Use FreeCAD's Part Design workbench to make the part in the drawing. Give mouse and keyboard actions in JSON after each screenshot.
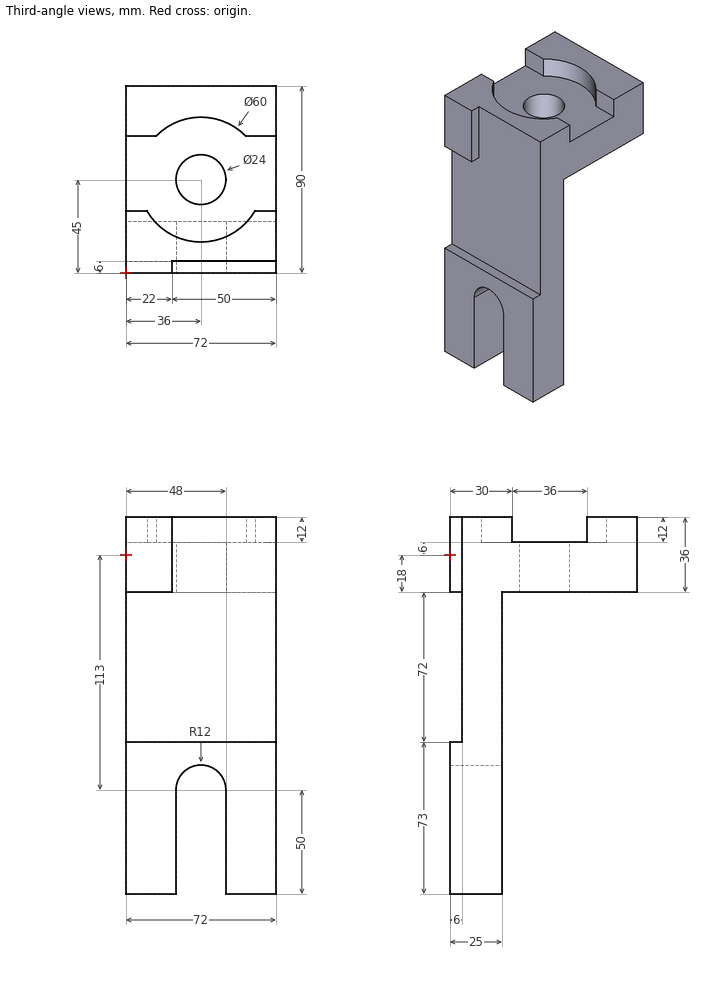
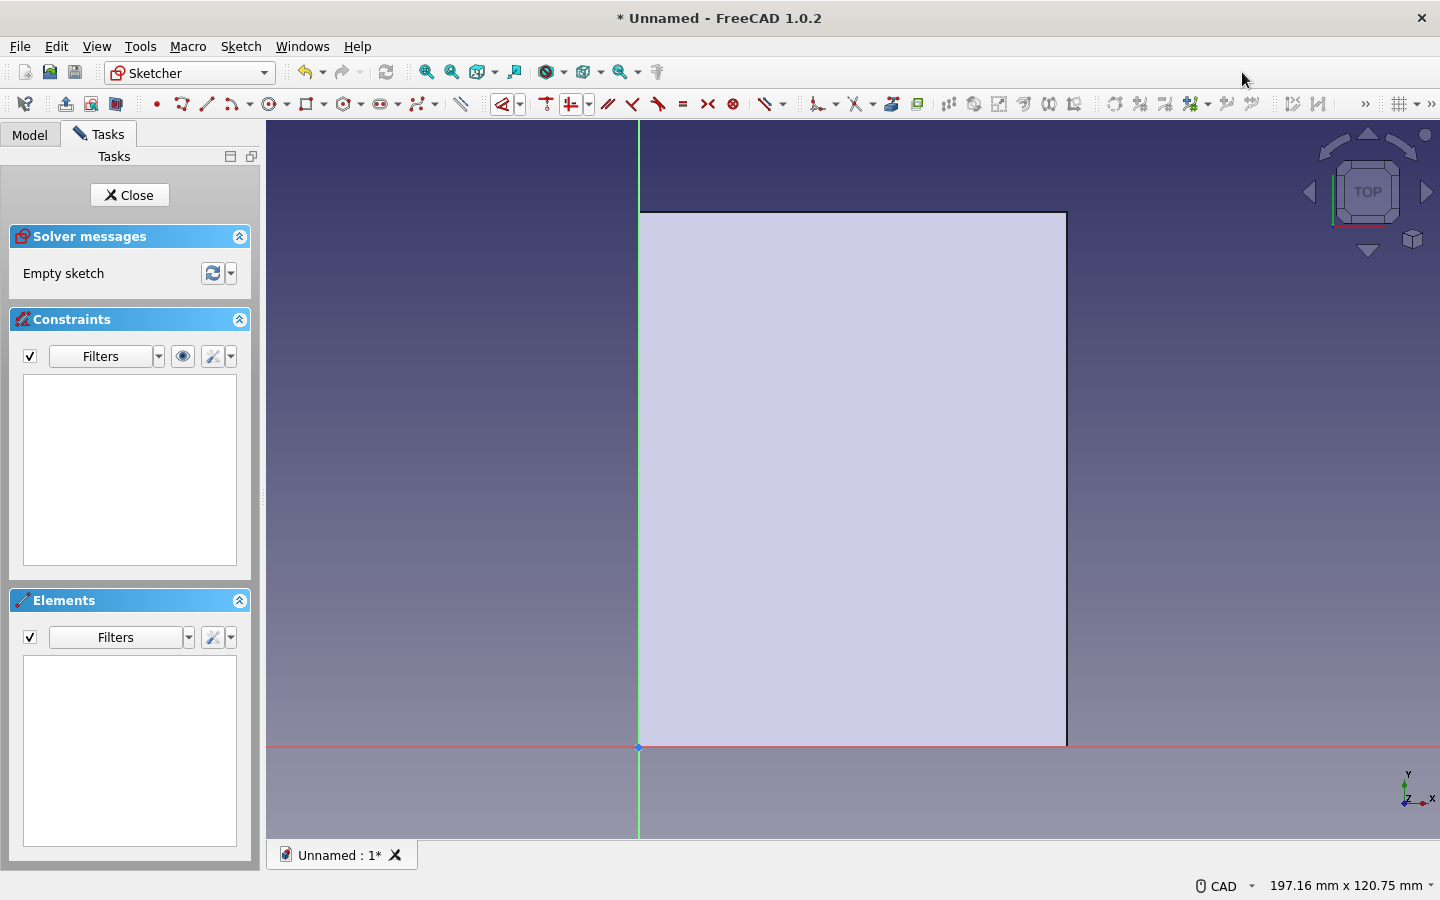
{"action": "key", "text": "g c"}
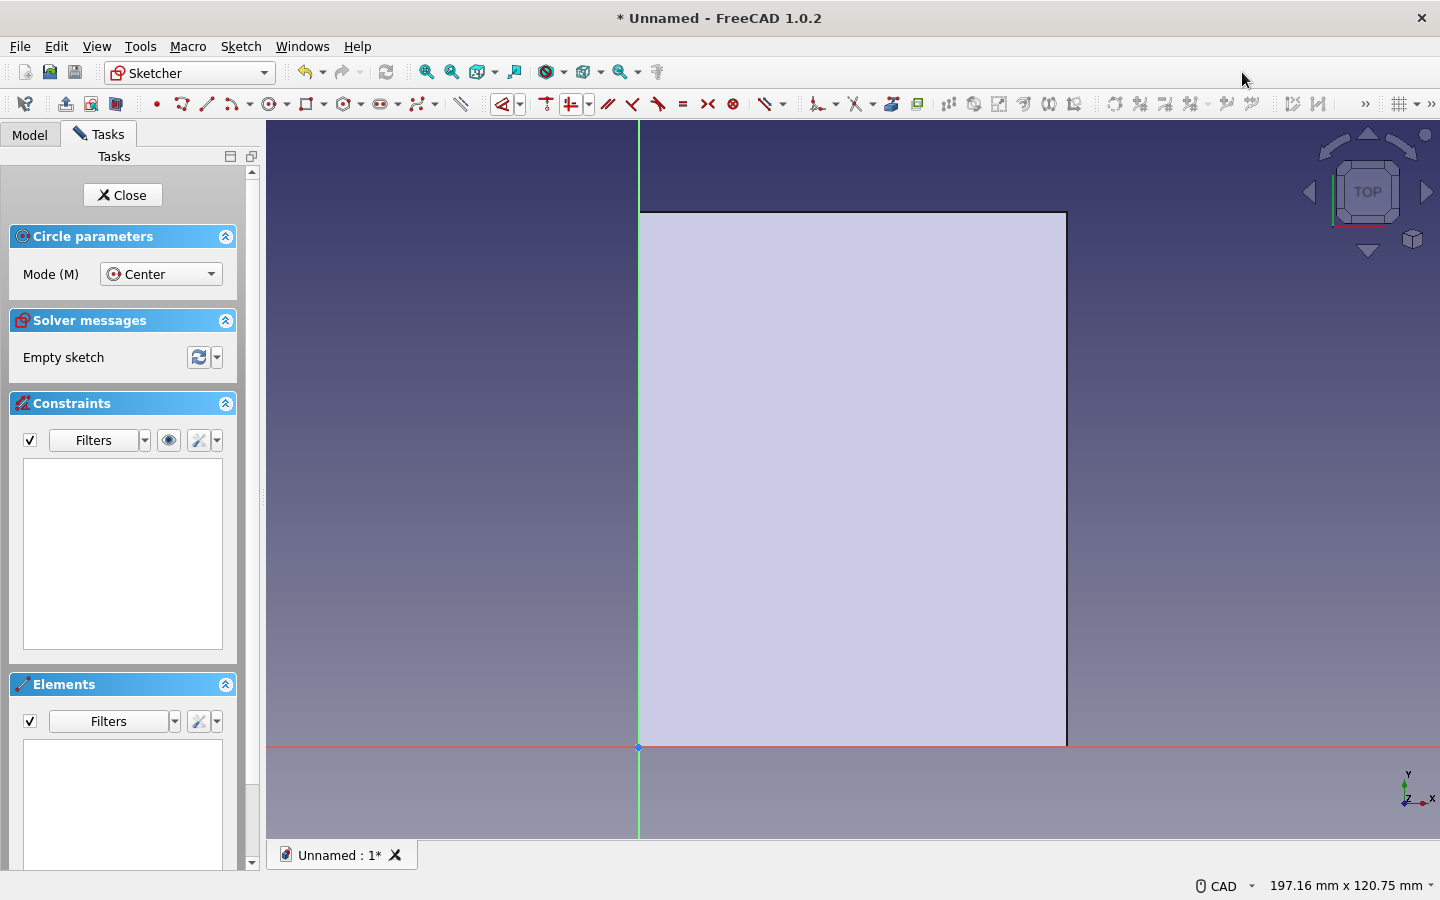
{"action": "left_click", "coordinate": [853, 480]}
{"action": "mouse_move", "coordinate": [979, 353]}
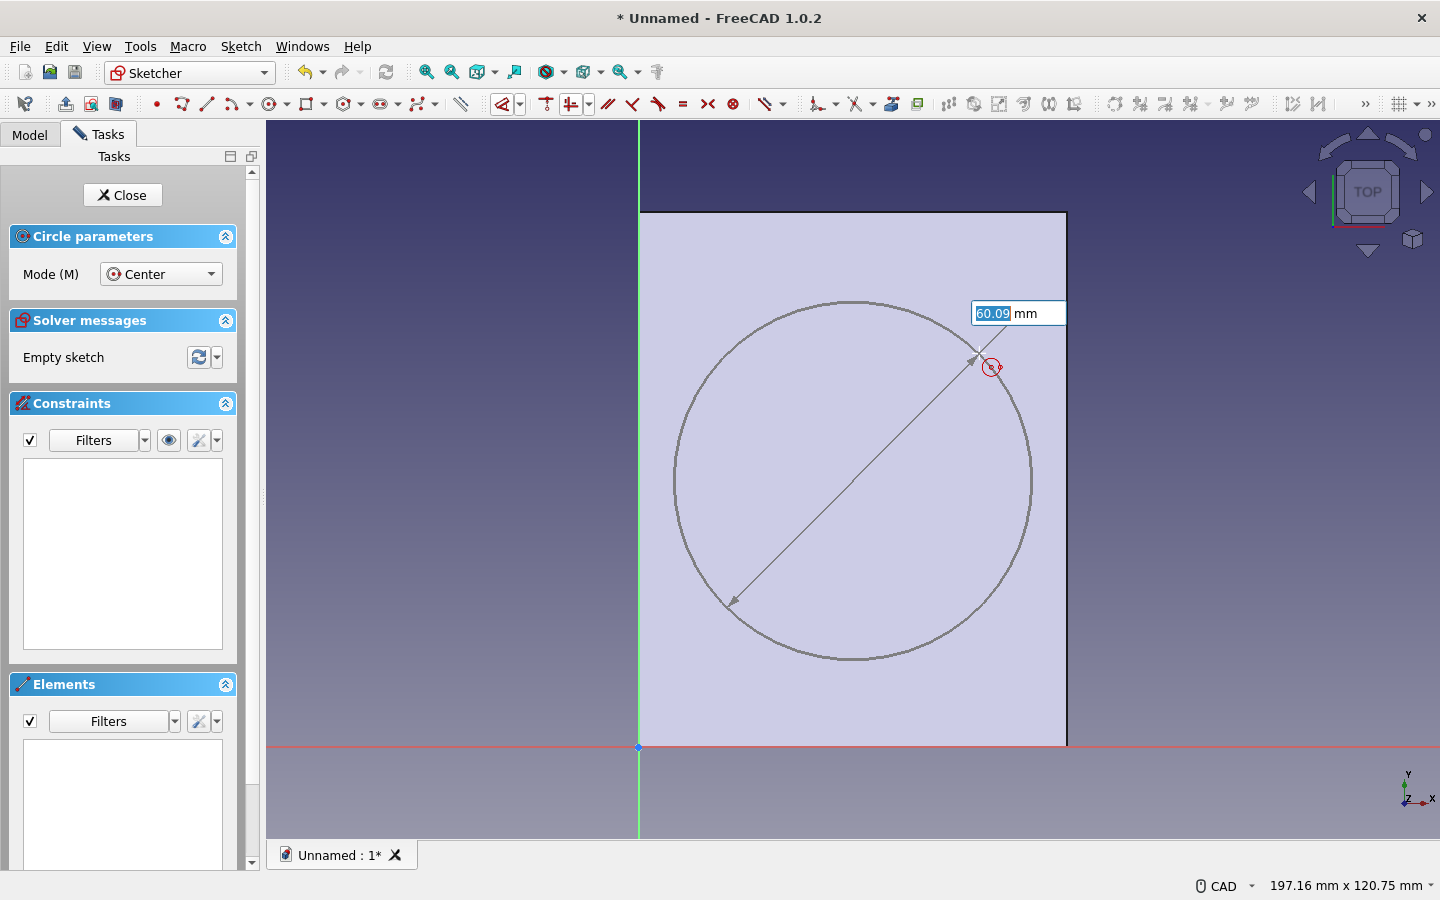
{"action": "type", "text": "60"}
{"action": "key", "text": "Return"}
{"action": "key", "text": "Escape"}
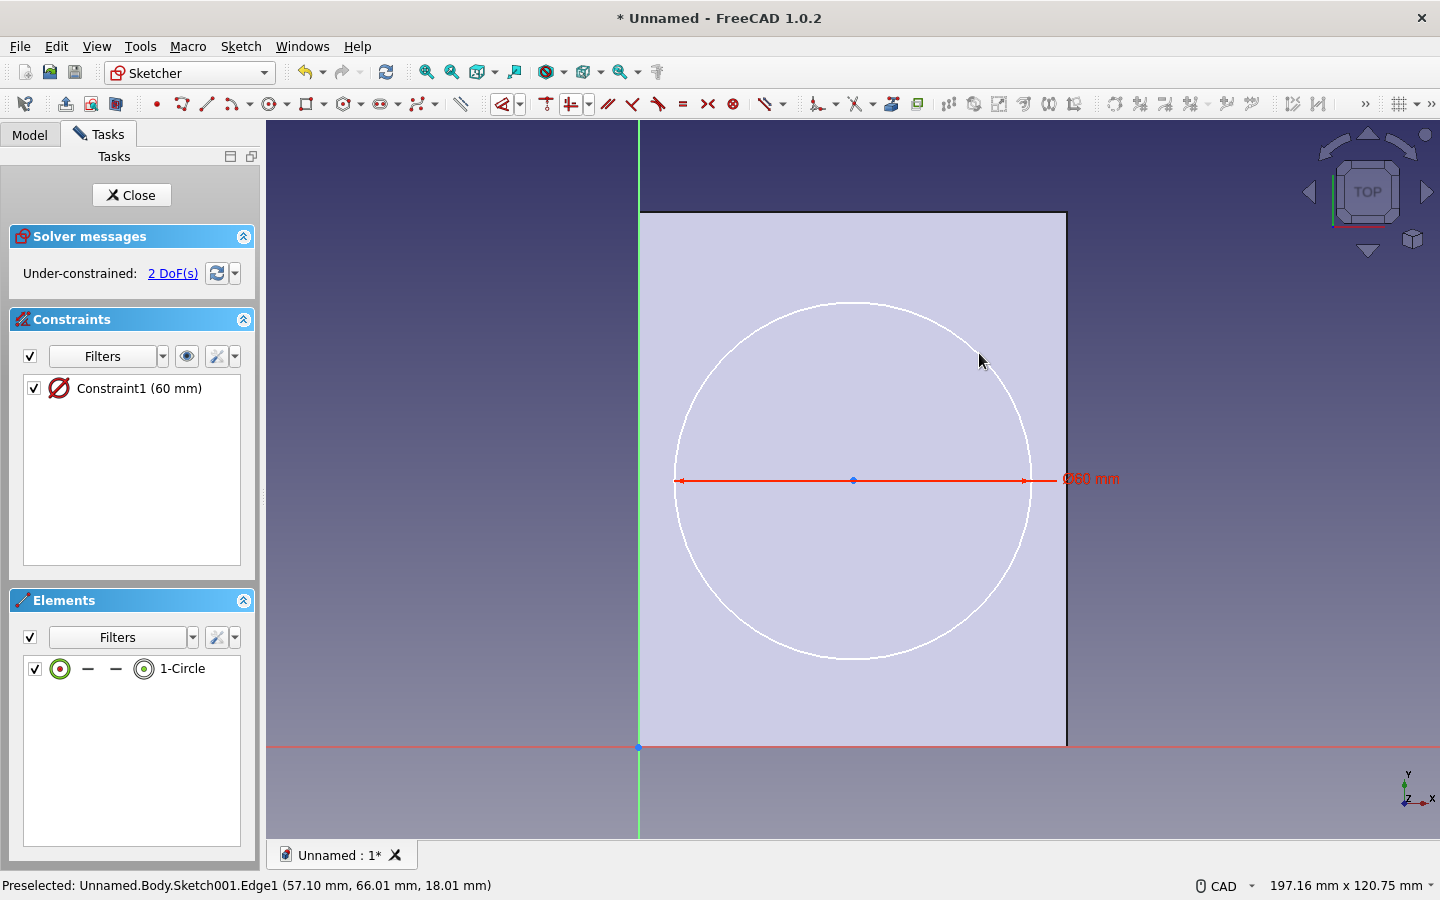
{"action": "key", "text": "d"}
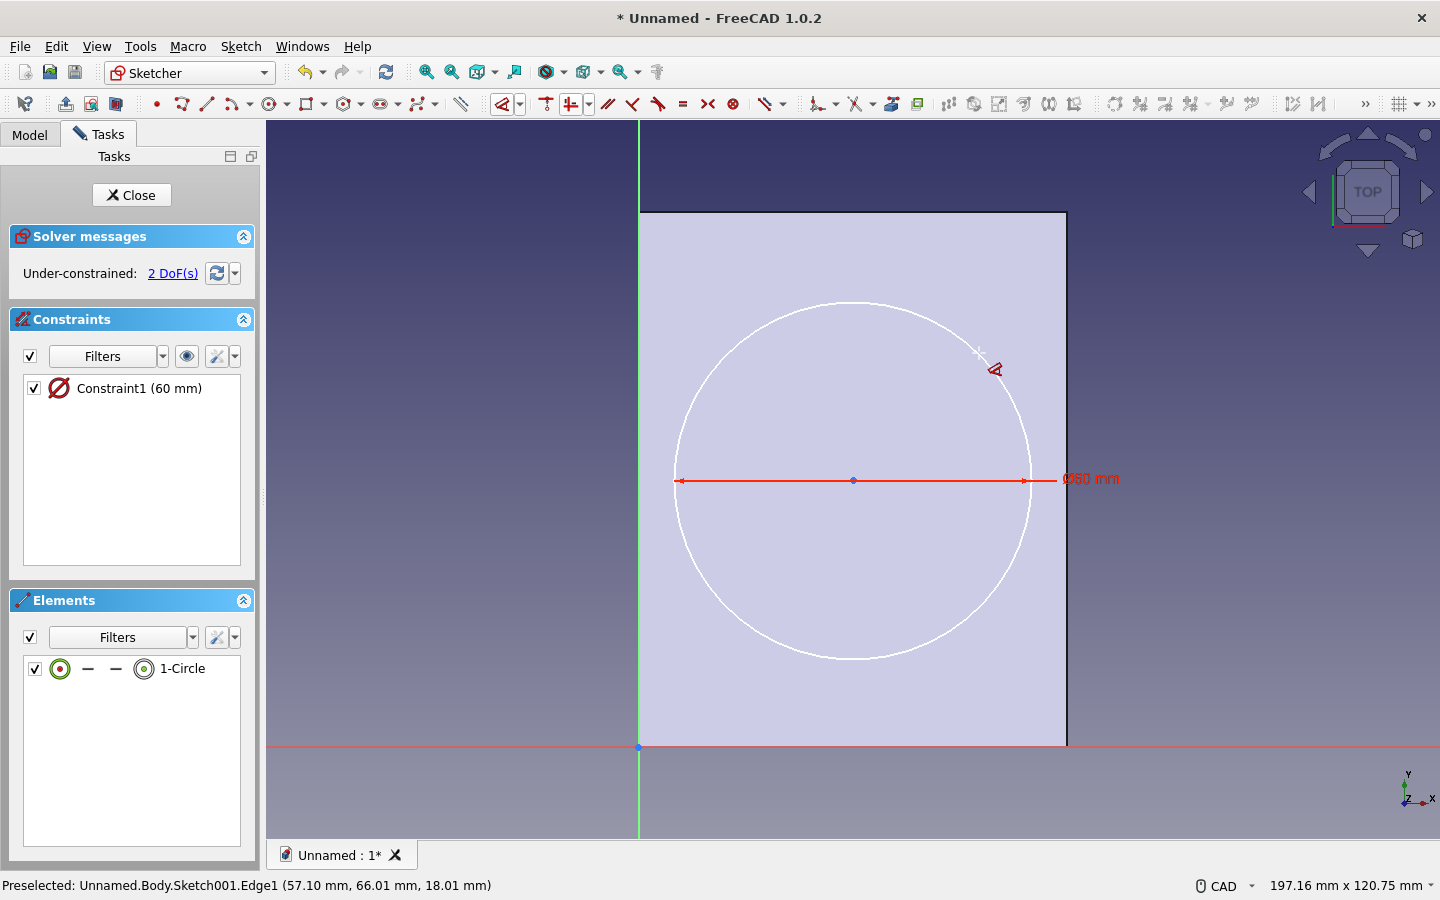
{"action": "left_click", "coordinate": [853, 481]}
{"action": "left_click", "coordinate": [746, 781]}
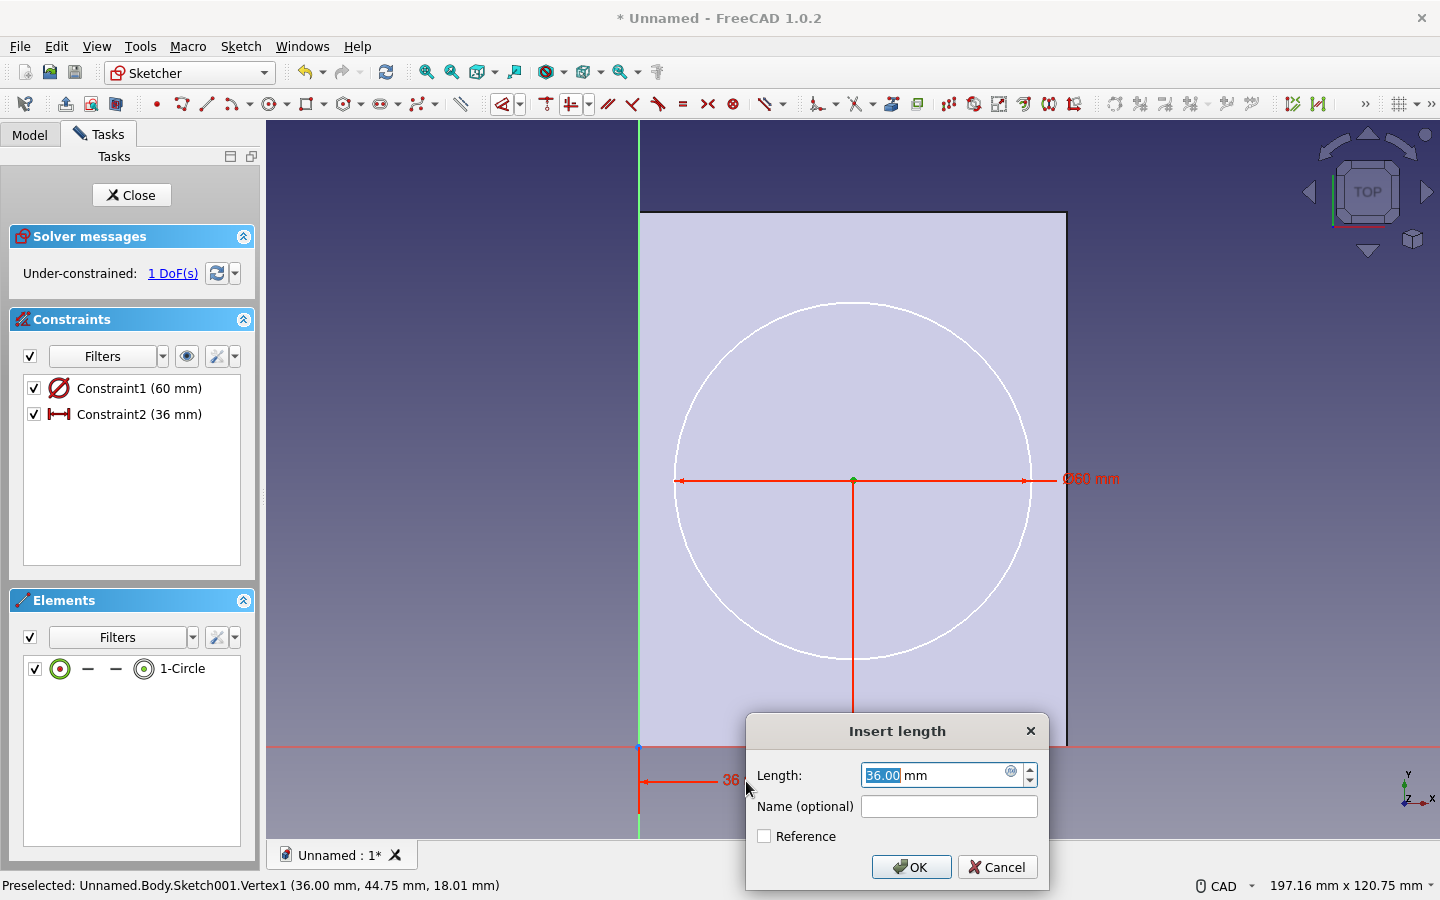
{"action": "type", "text": "36"}
{"action": "key", "text": "Return"}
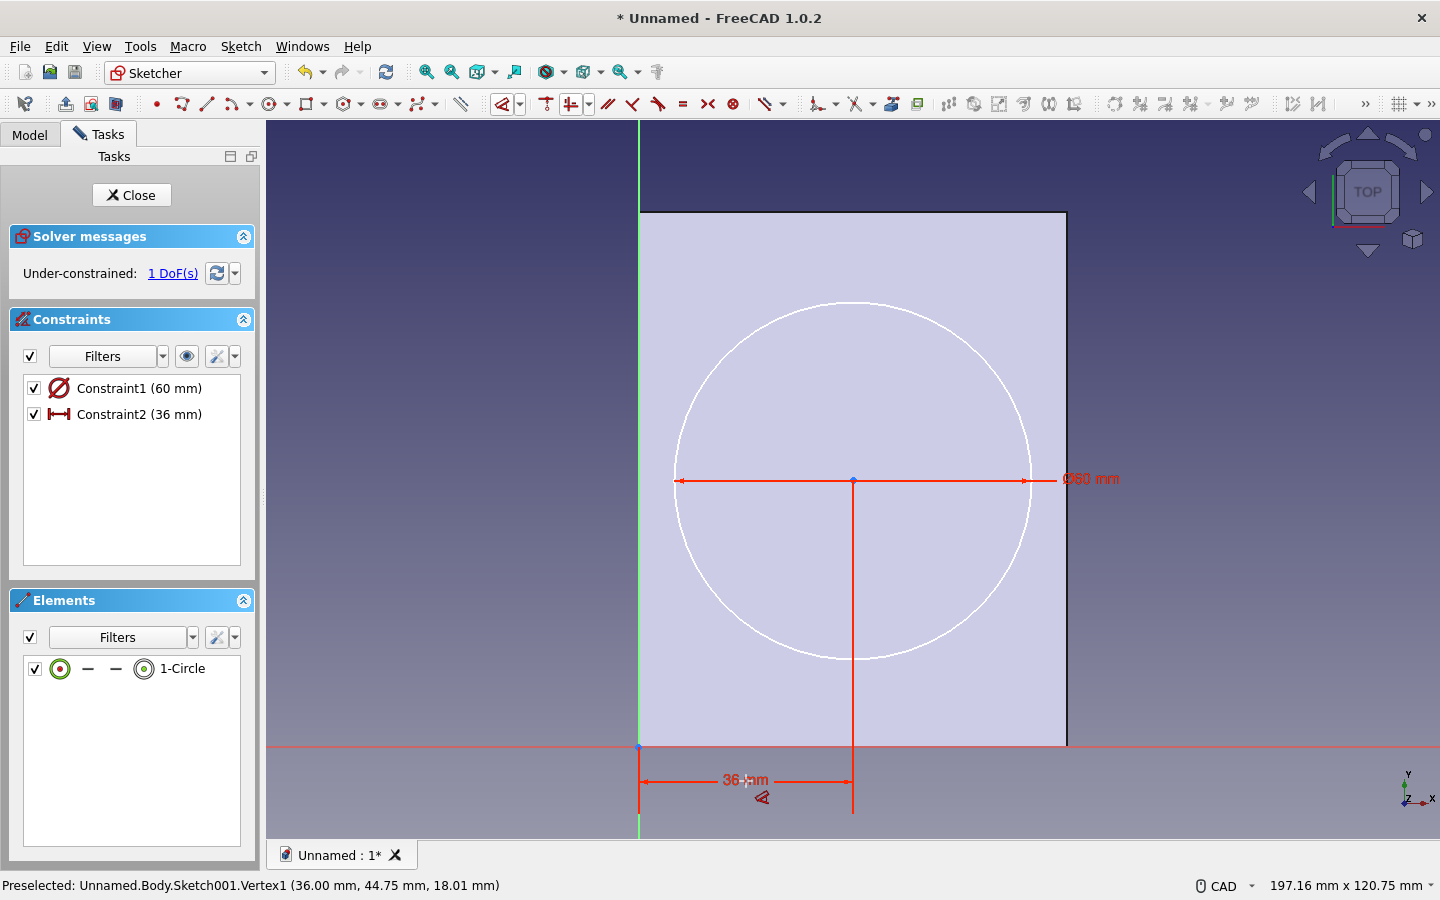
{"action": "left_click", "coordinate": [853, 481]}
{"action": "left_click", "coordinate": [605, 614]}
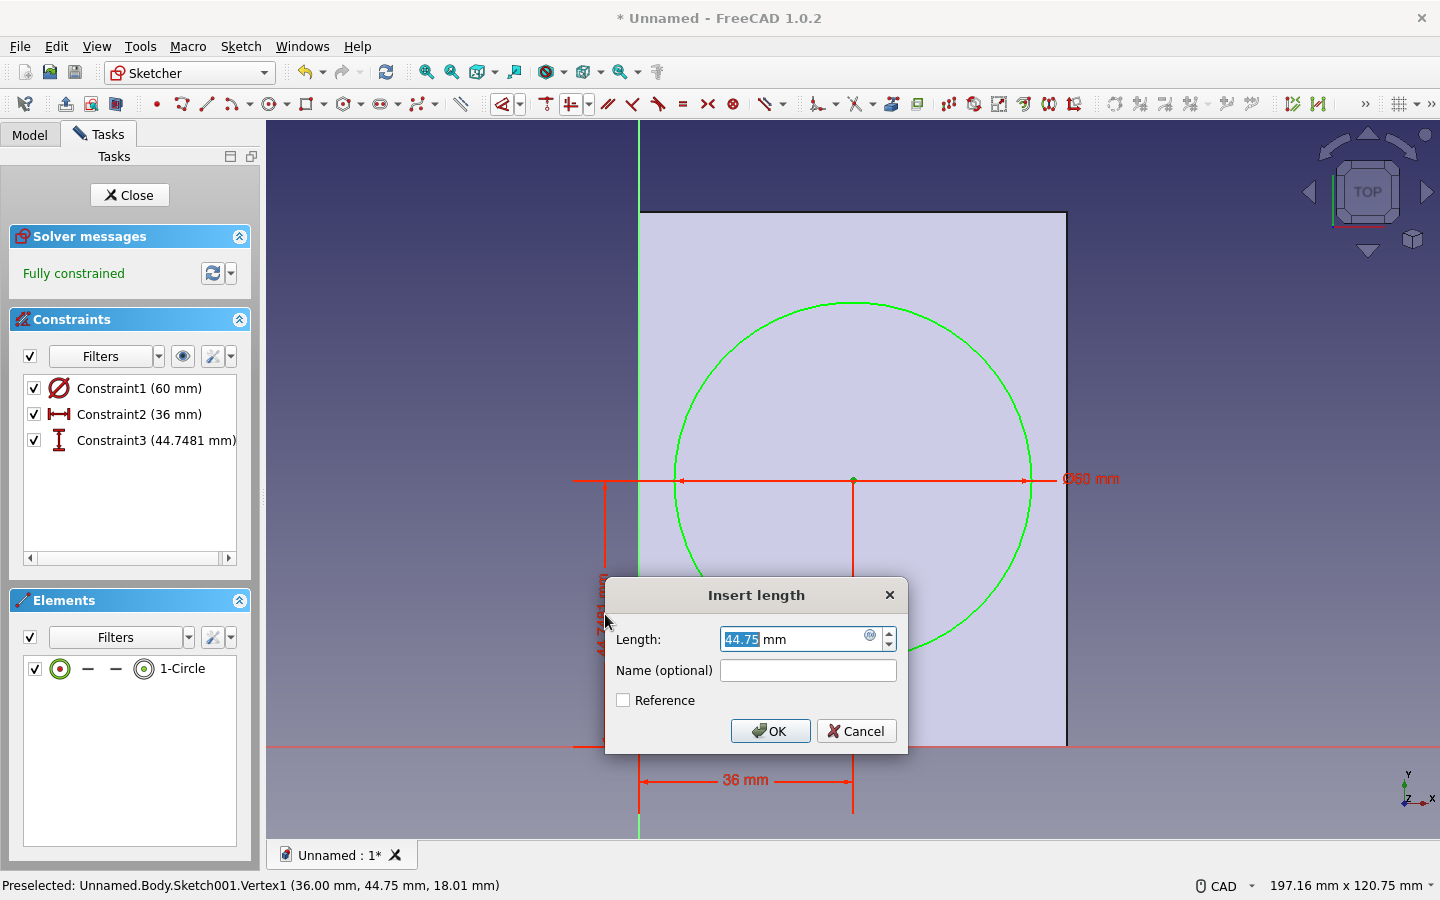
{"action": "type", "text": "45"}
{"action": "key", "text": "Return"}
{"action": "key", "text": "Escape"}